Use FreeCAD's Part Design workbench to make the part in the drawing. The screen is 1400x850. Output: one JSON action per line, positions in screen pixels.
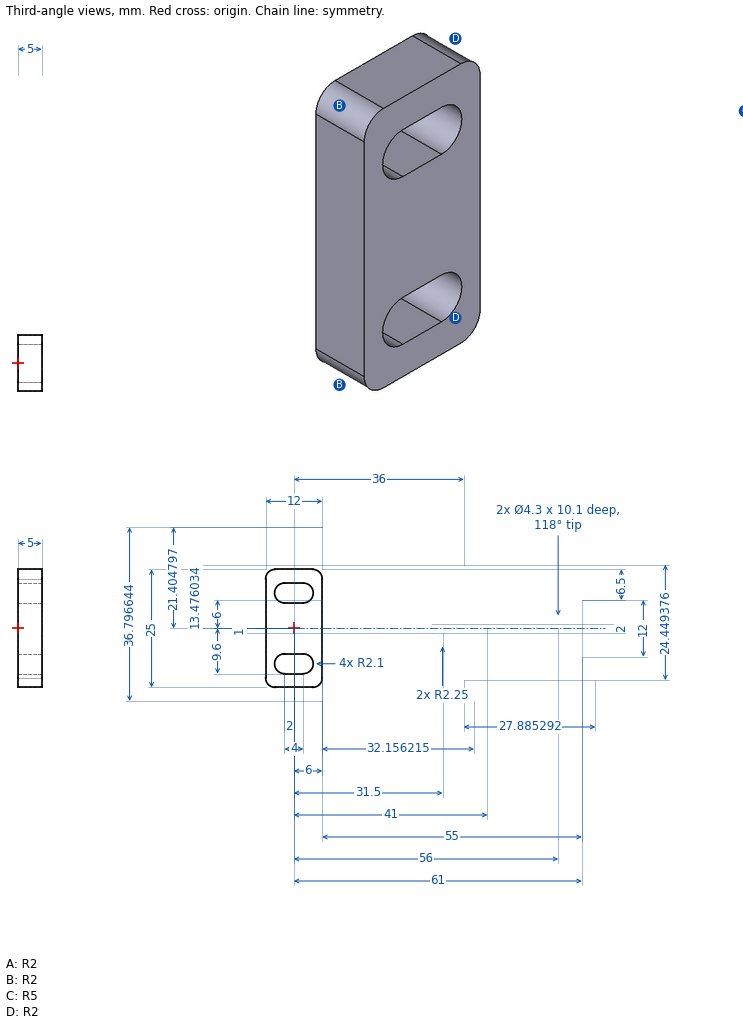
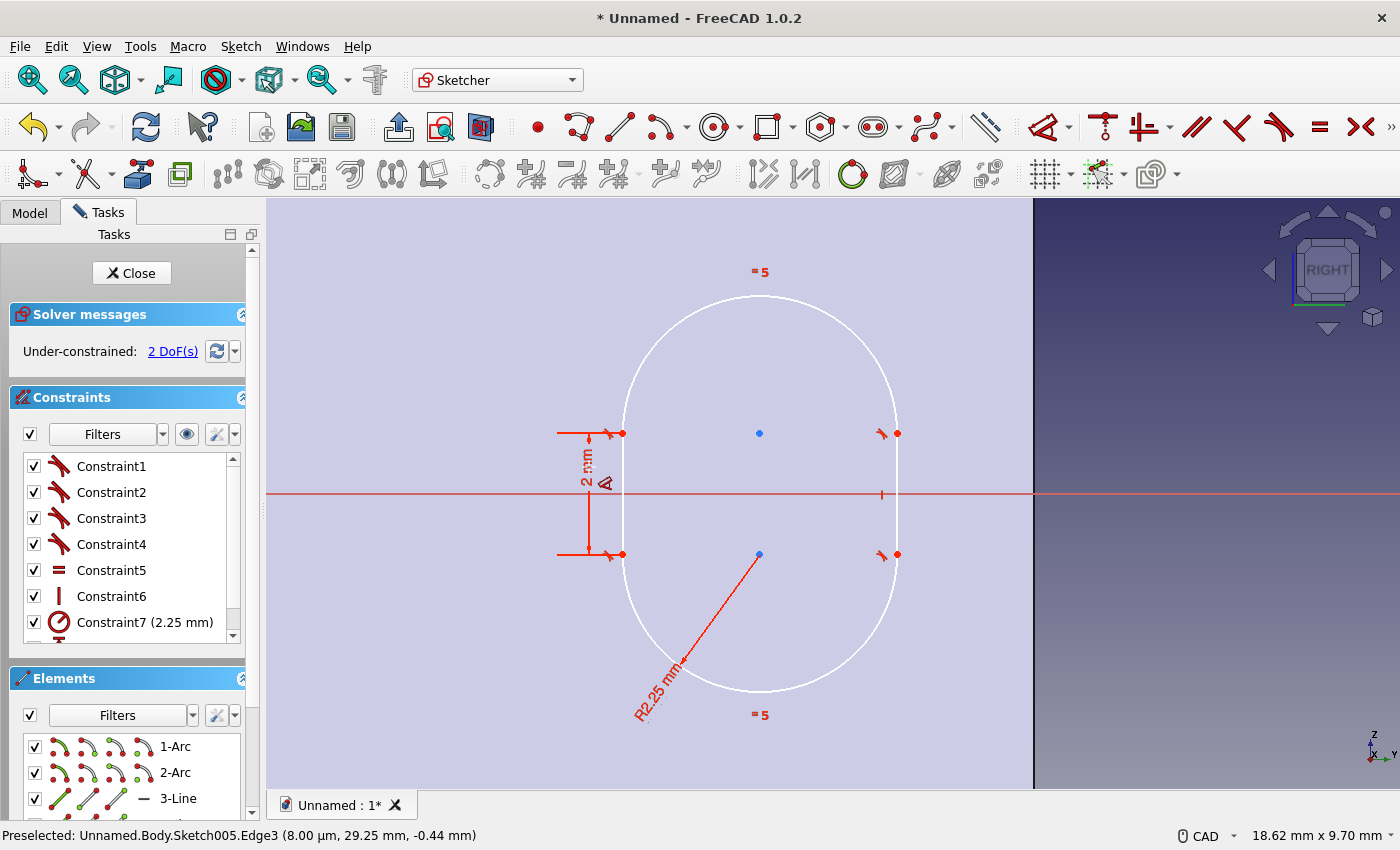
{"action": "left_click", "coordinate": [623, 555]}
{"action": "left_click", "coordinate": [657, 524]}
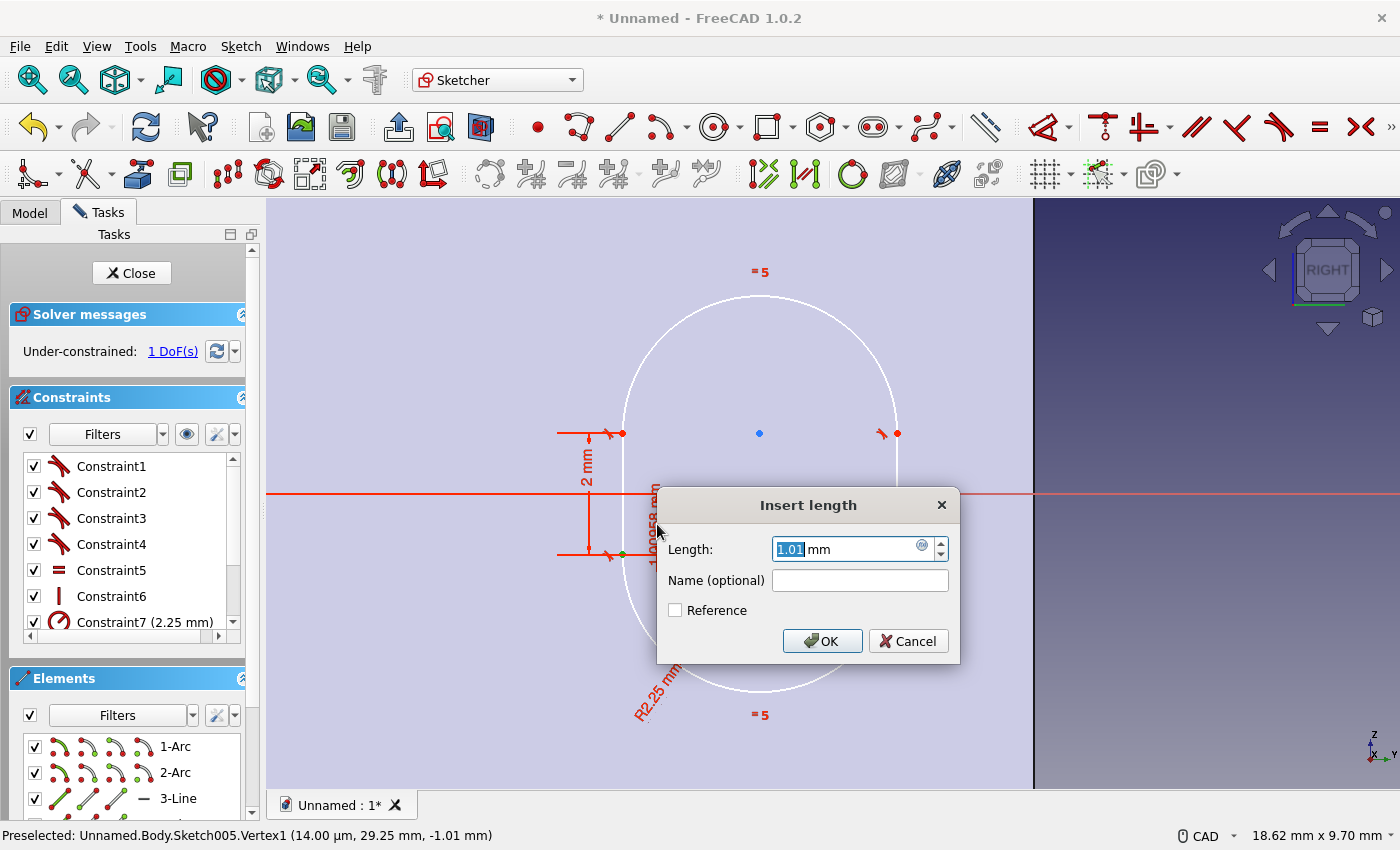
{"action": "type", "text": "1"}
{"action": "key", "text": "Return"}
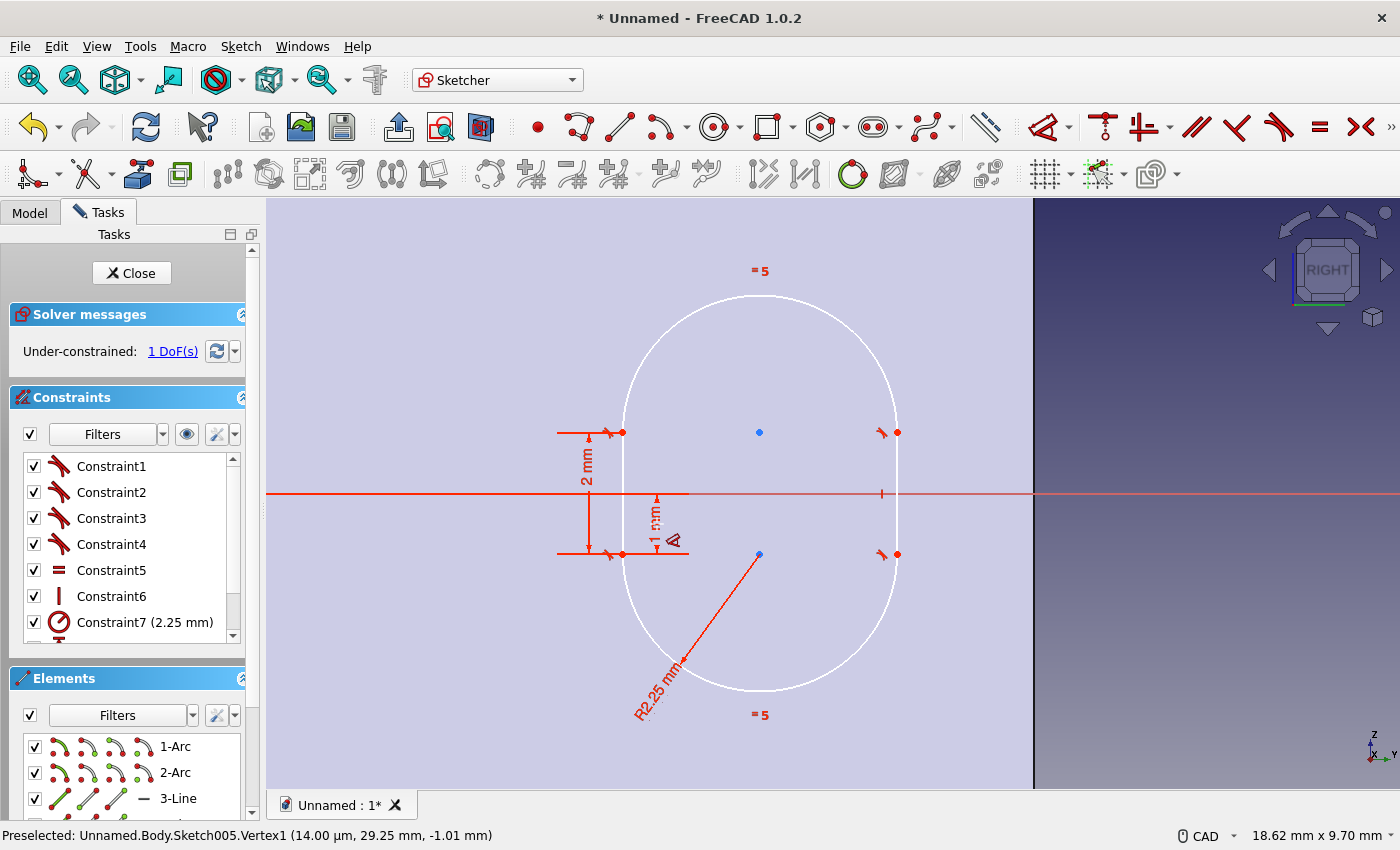
{"action": "left_click", "coordinate": [760, 554]}
{"action": "left_click", "coordinate": [527, 588]}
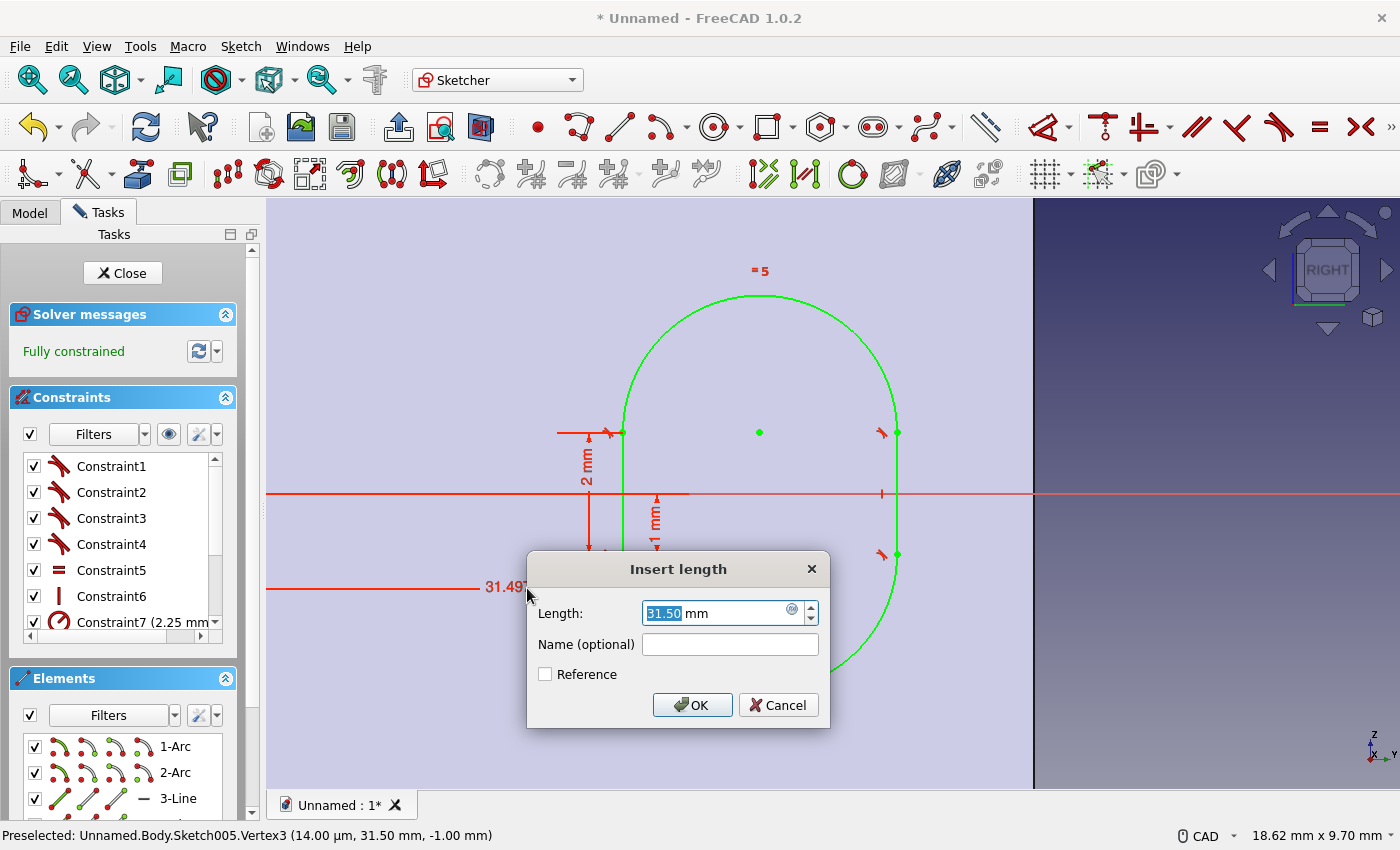
{"action": "type", "text": "31.5"}
{"action": "key", "text": "Return"}
{"action": "key", "text": "Escape"}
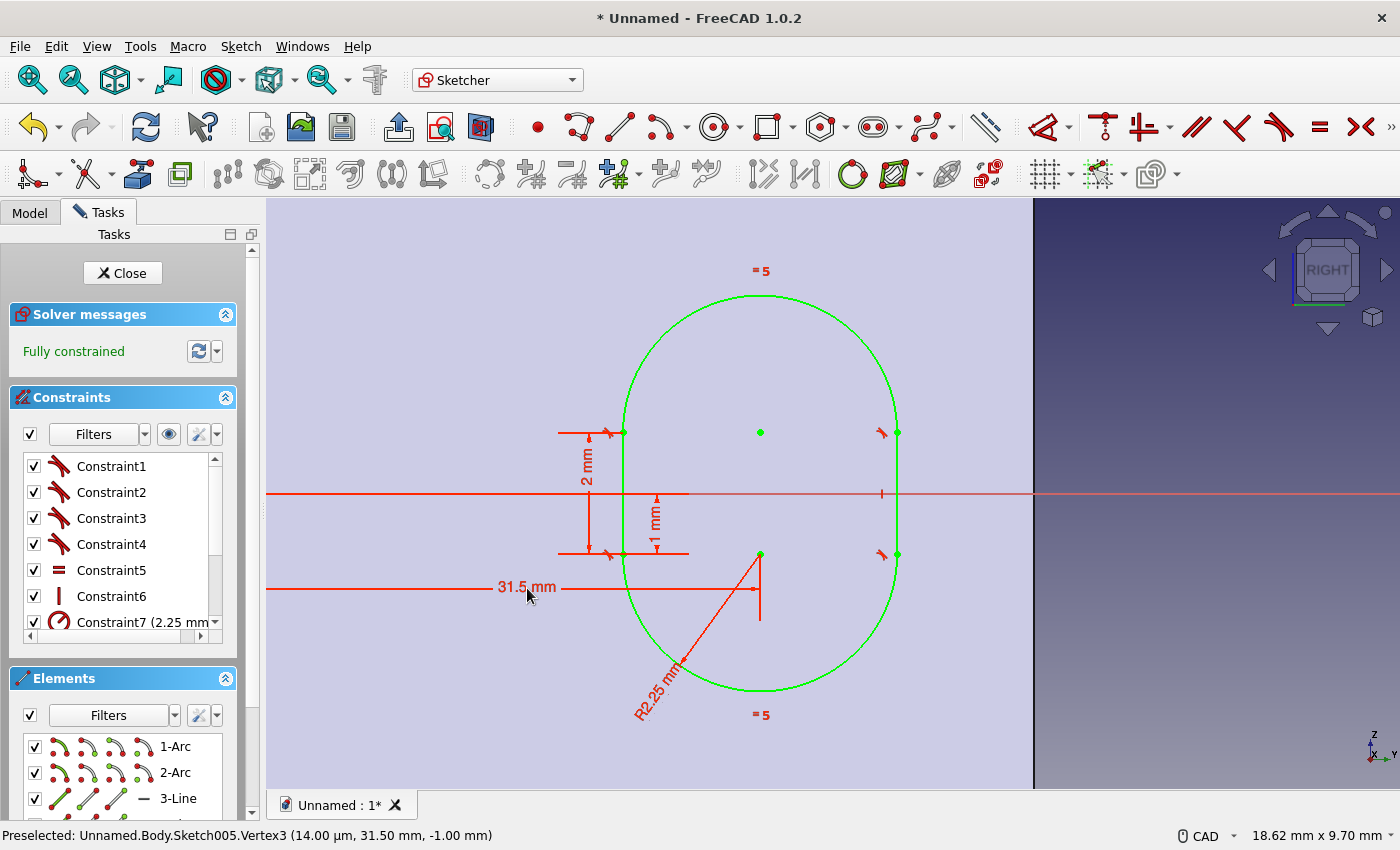
{"action": "left_click", "coordinate": [123, 273]}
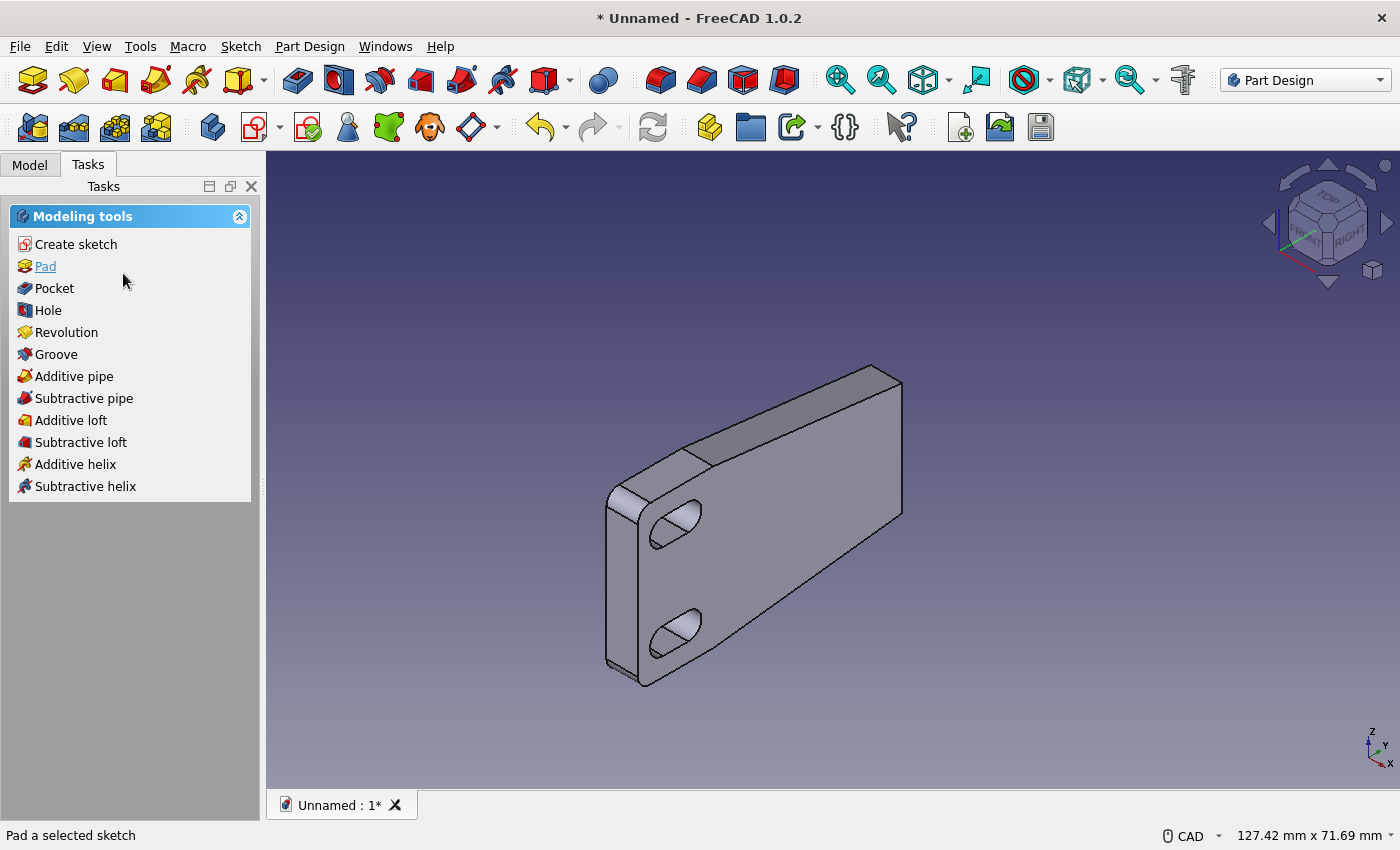
{"action": "left_click", "coordinate": [298, 80]}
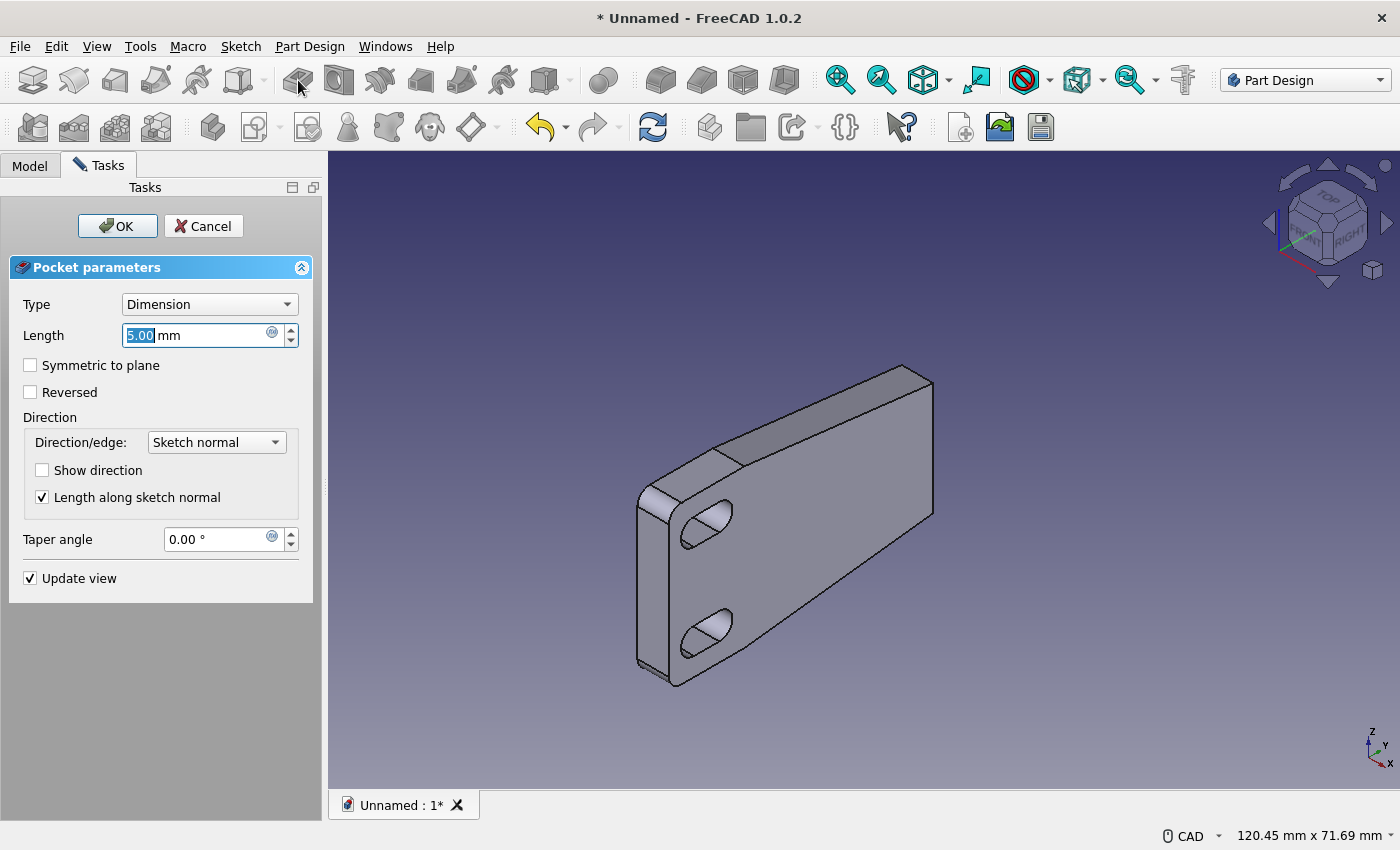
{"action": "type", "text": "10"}
{"action": "key", "text": "Tab"}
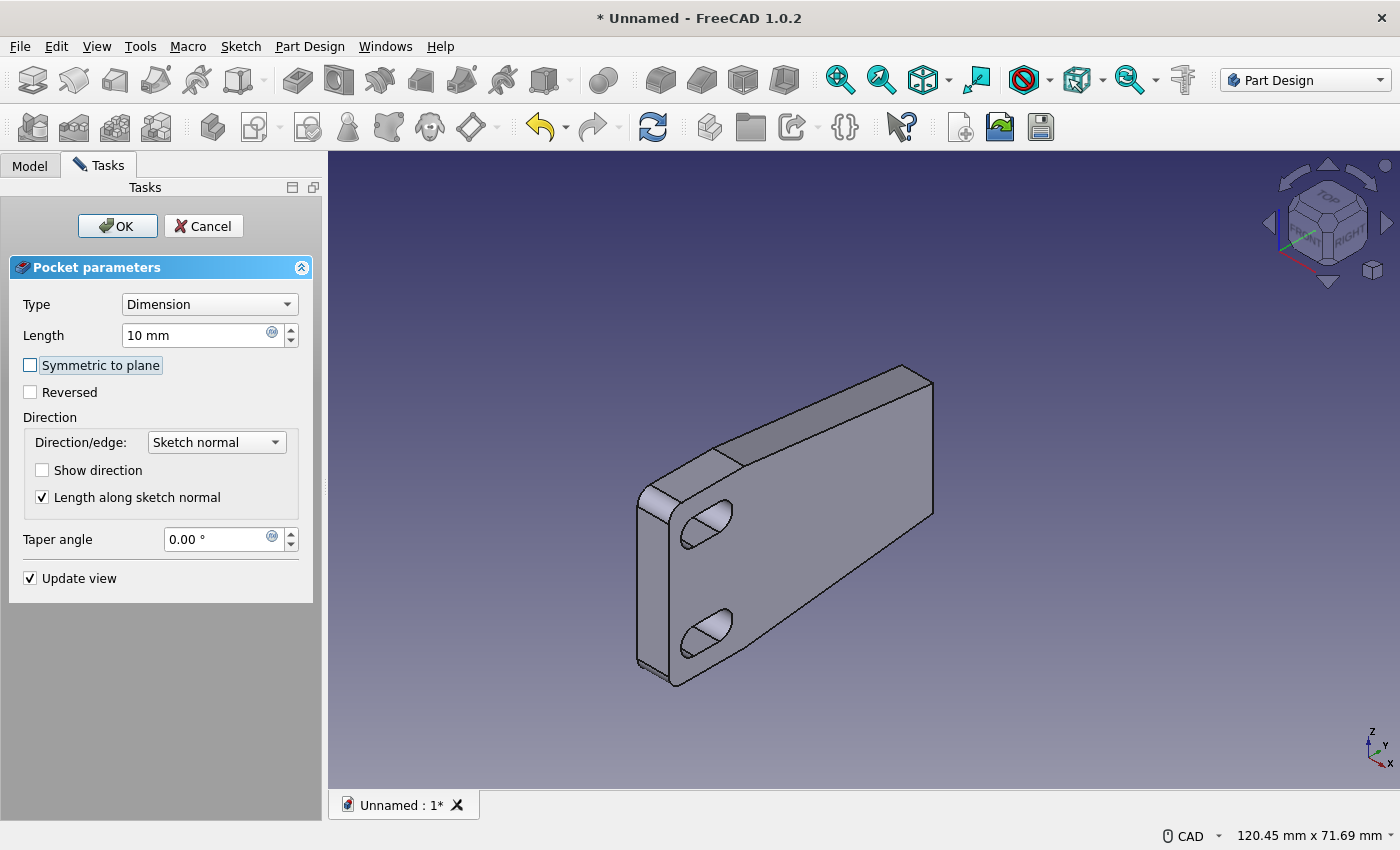
{"action": "left_click", "coordinate": [31, 392]}